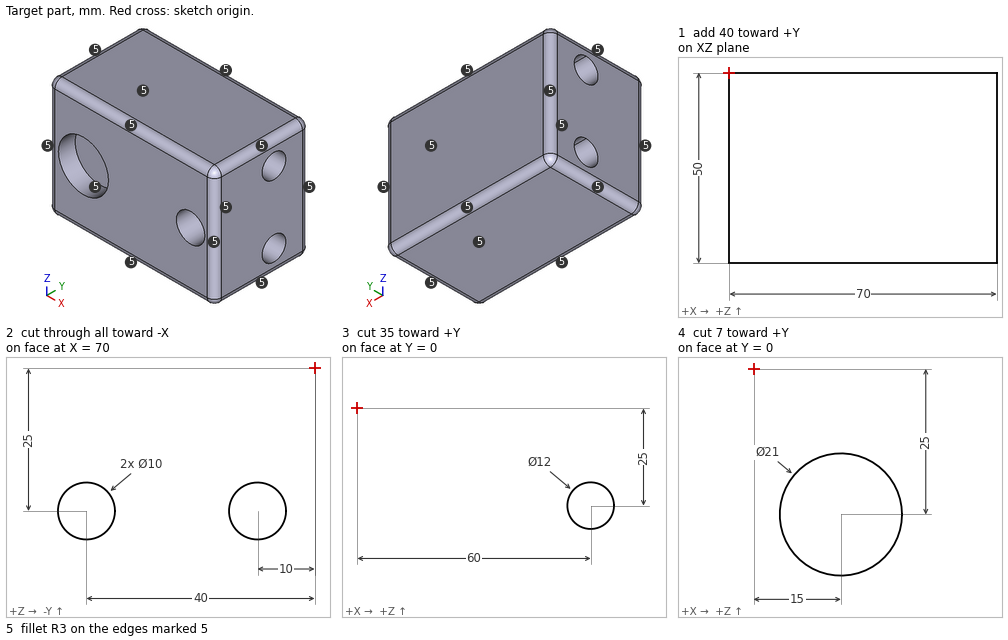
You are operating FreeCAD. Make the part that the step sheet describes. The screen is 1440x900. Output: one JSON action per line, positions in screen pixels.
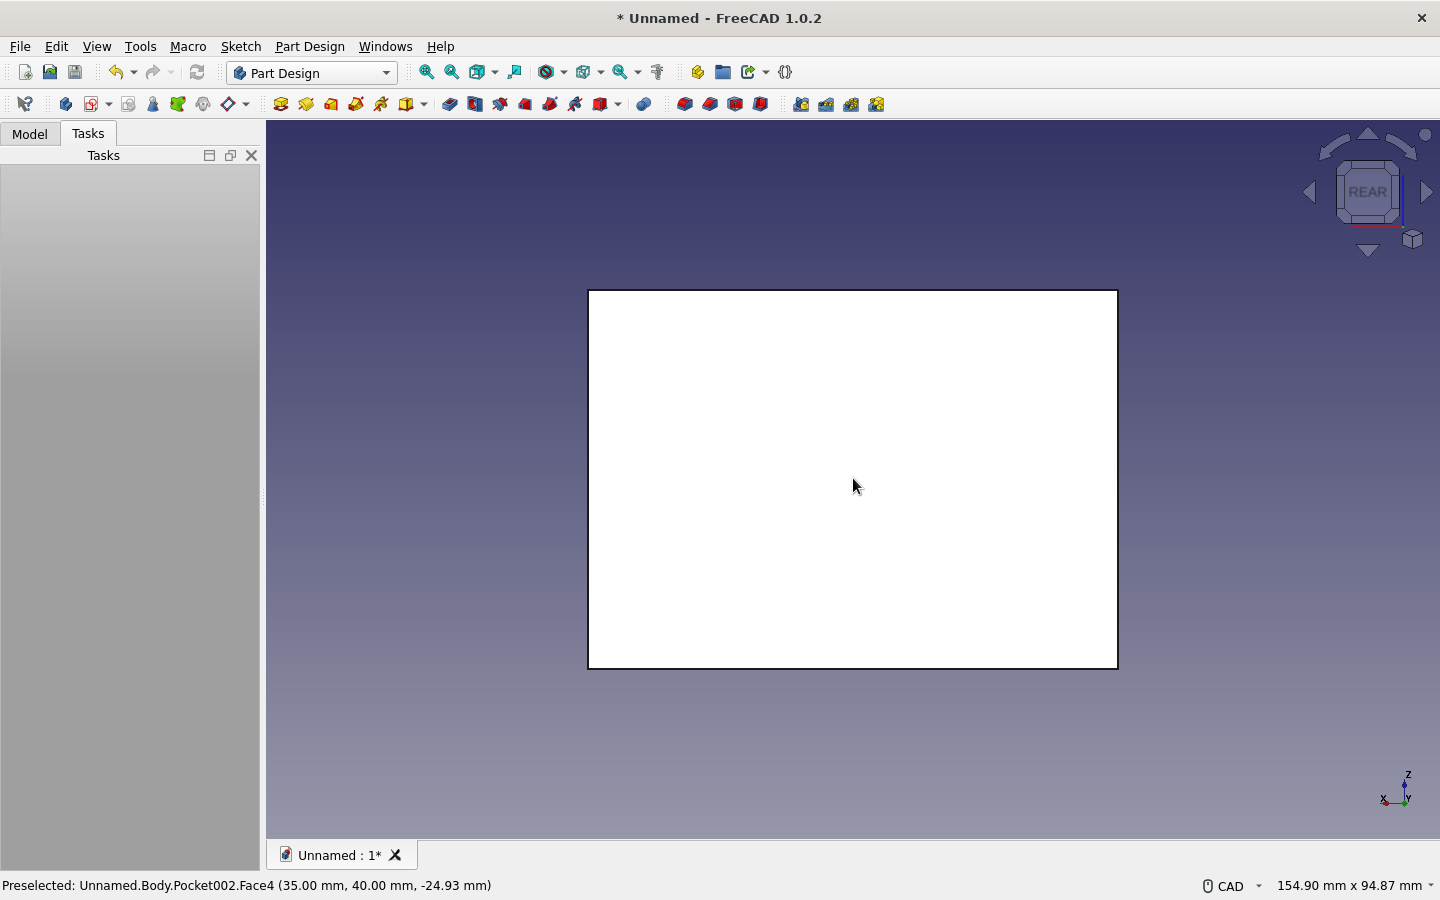
{"action": "key", "text": "6"}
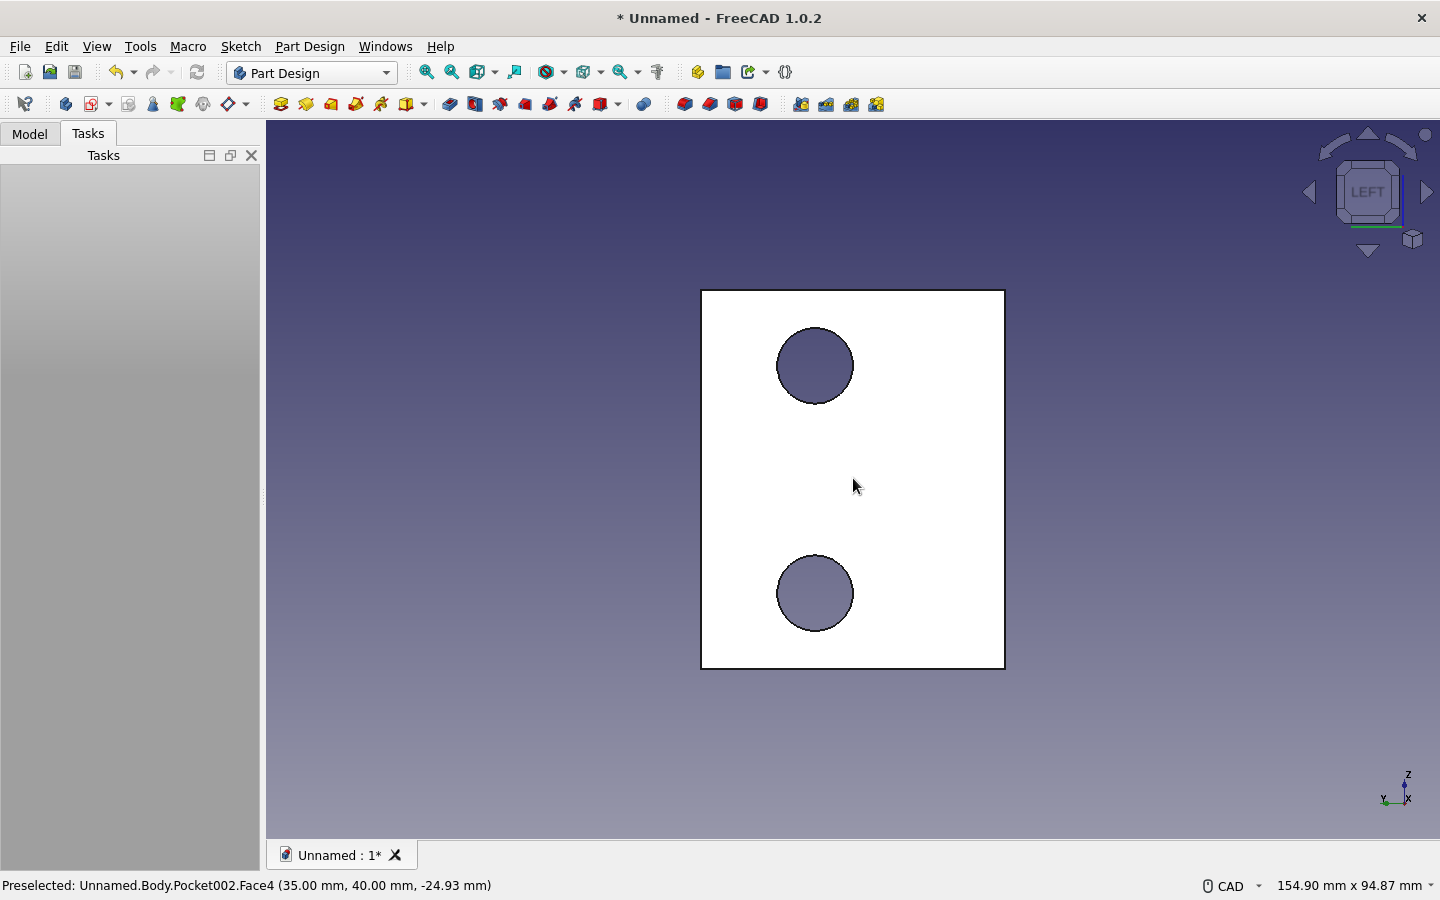
{"action": "key", "text": "v 3"}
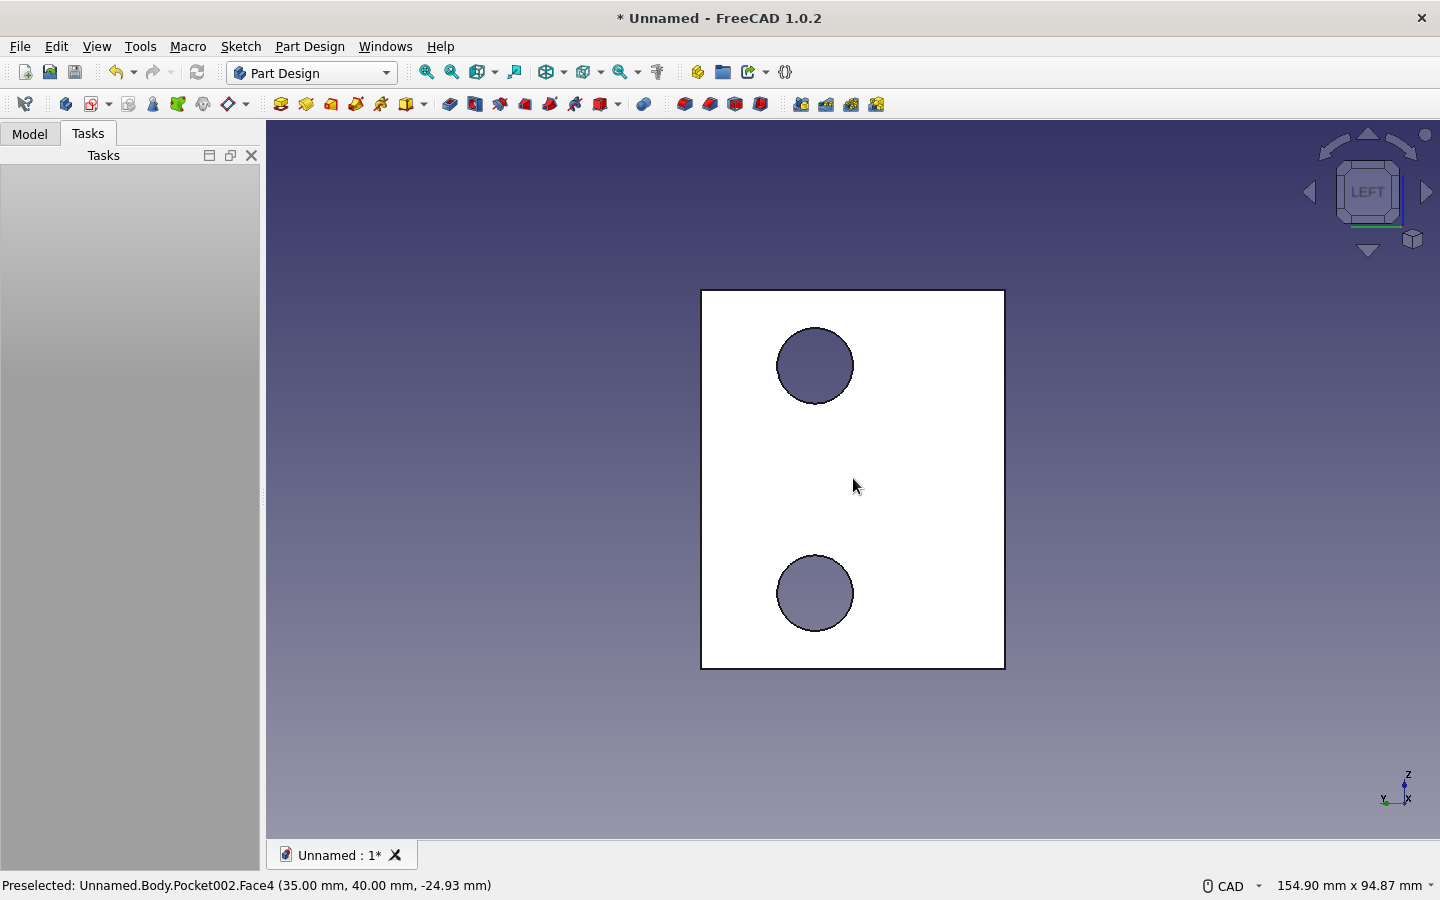
{"action": "key", "text": "0"}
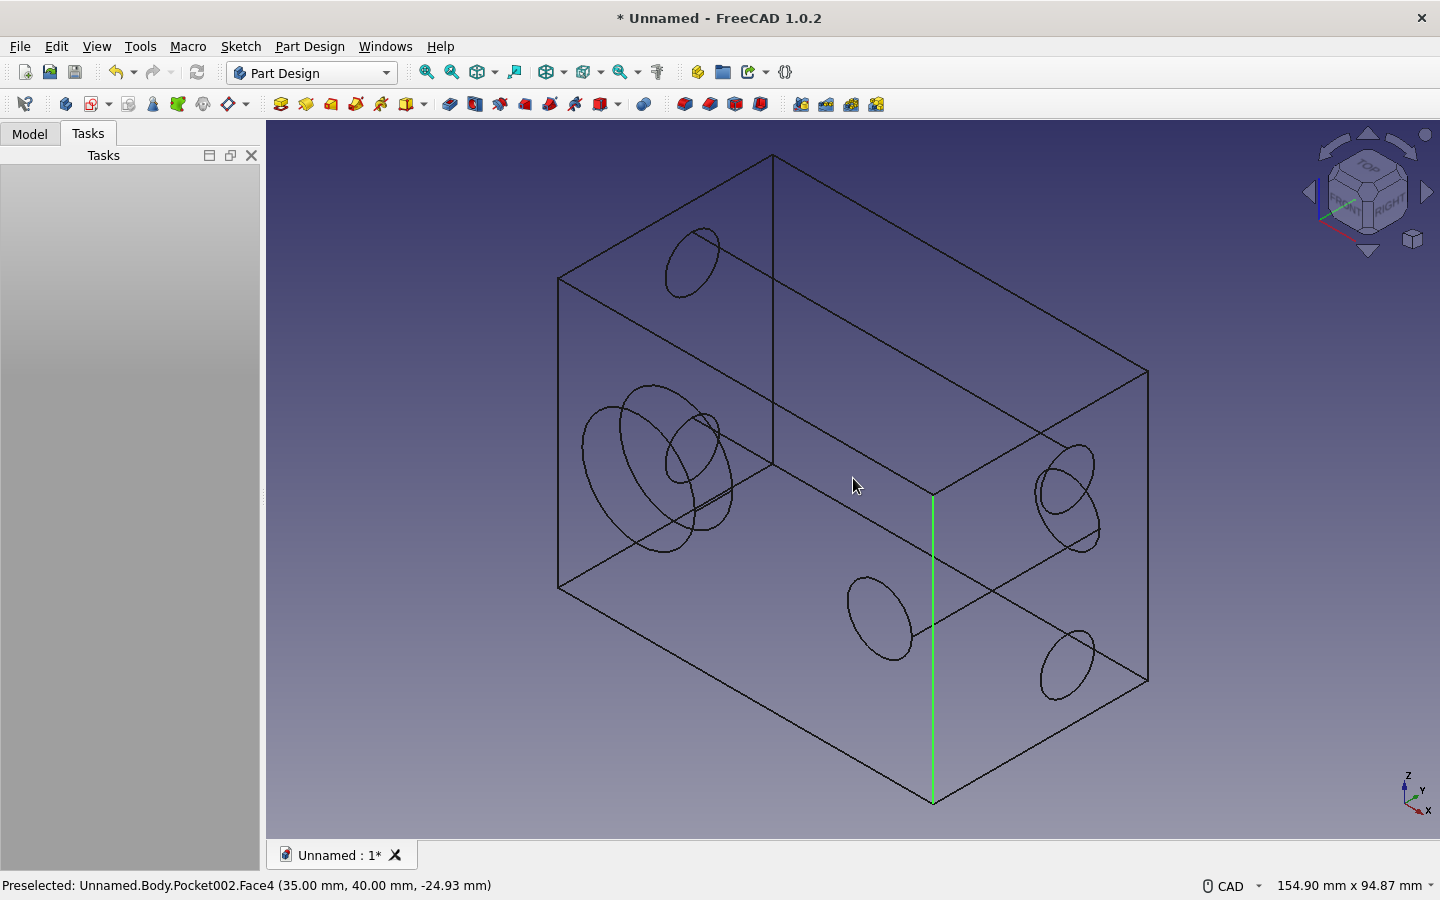
{"action": "left_click", "coordinate": [558, 432], "text": "ctrl"}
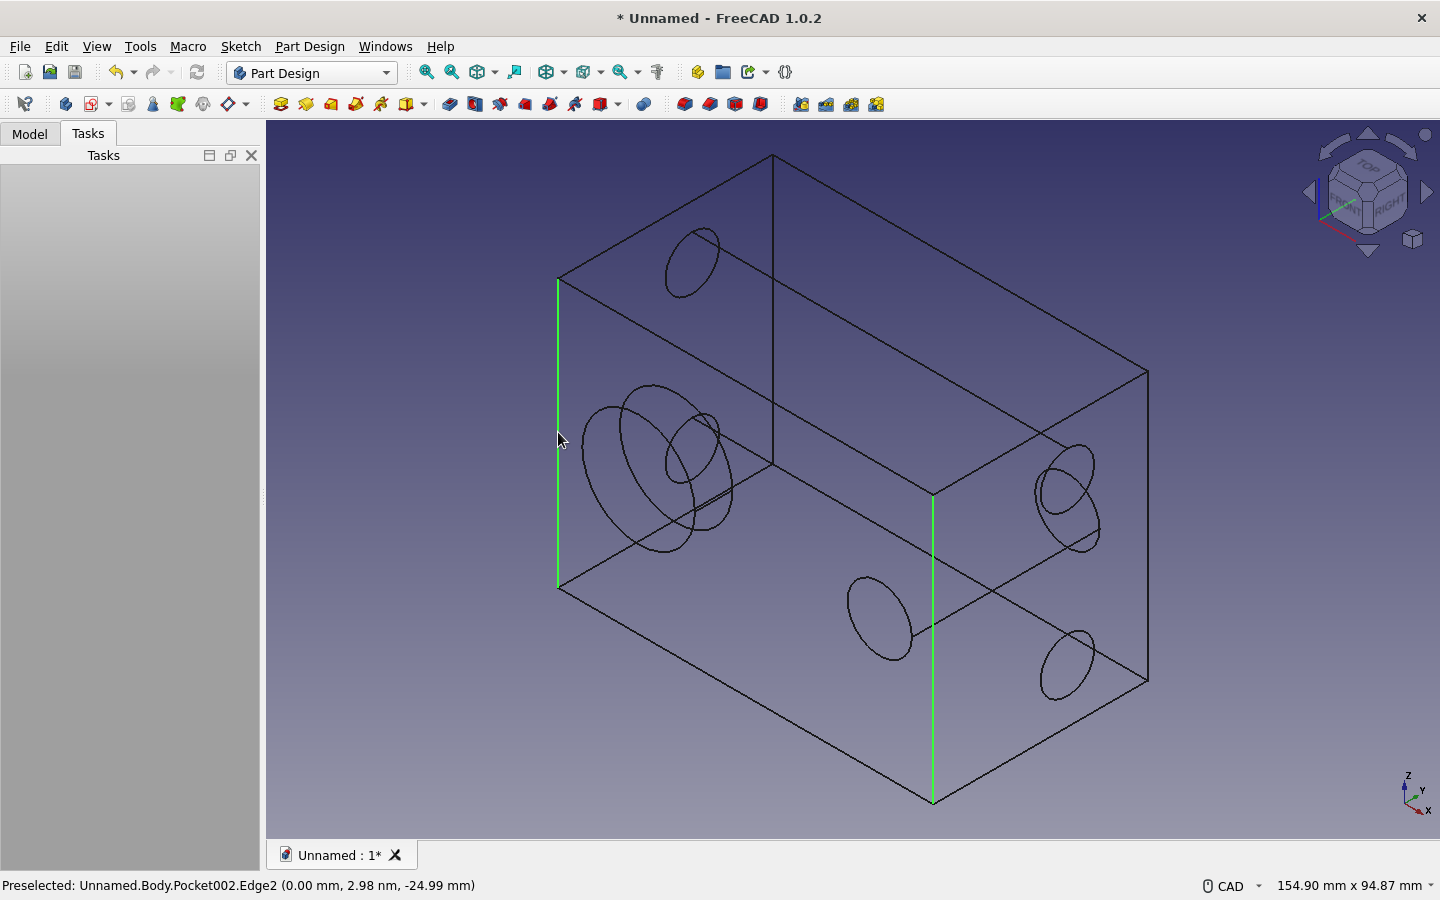
{"action": "key", "text": "v 1"}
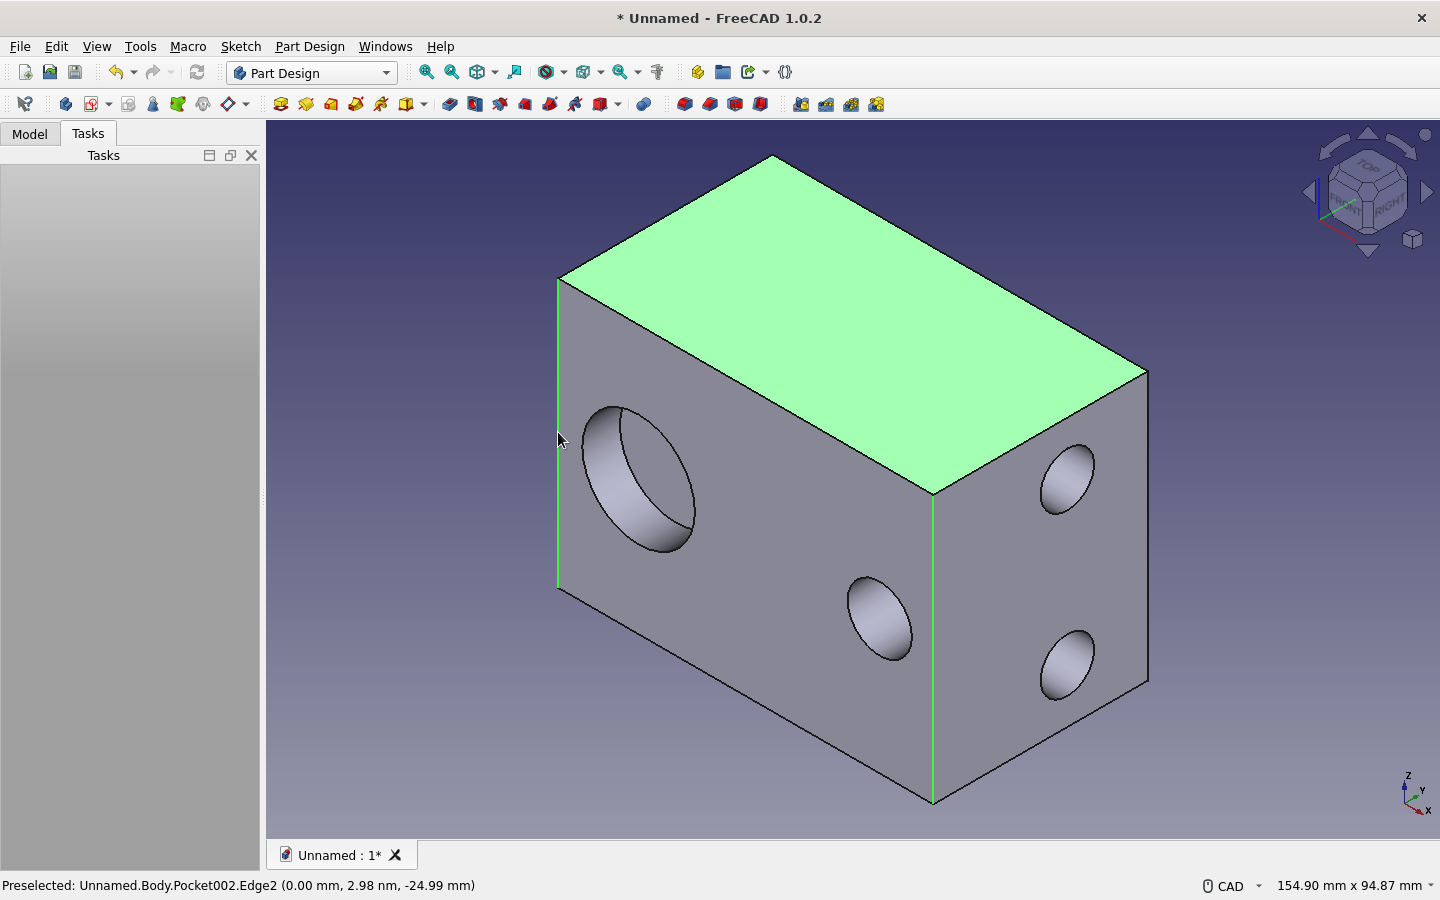
{"action": "left_click", "coordinate": [685, 104]}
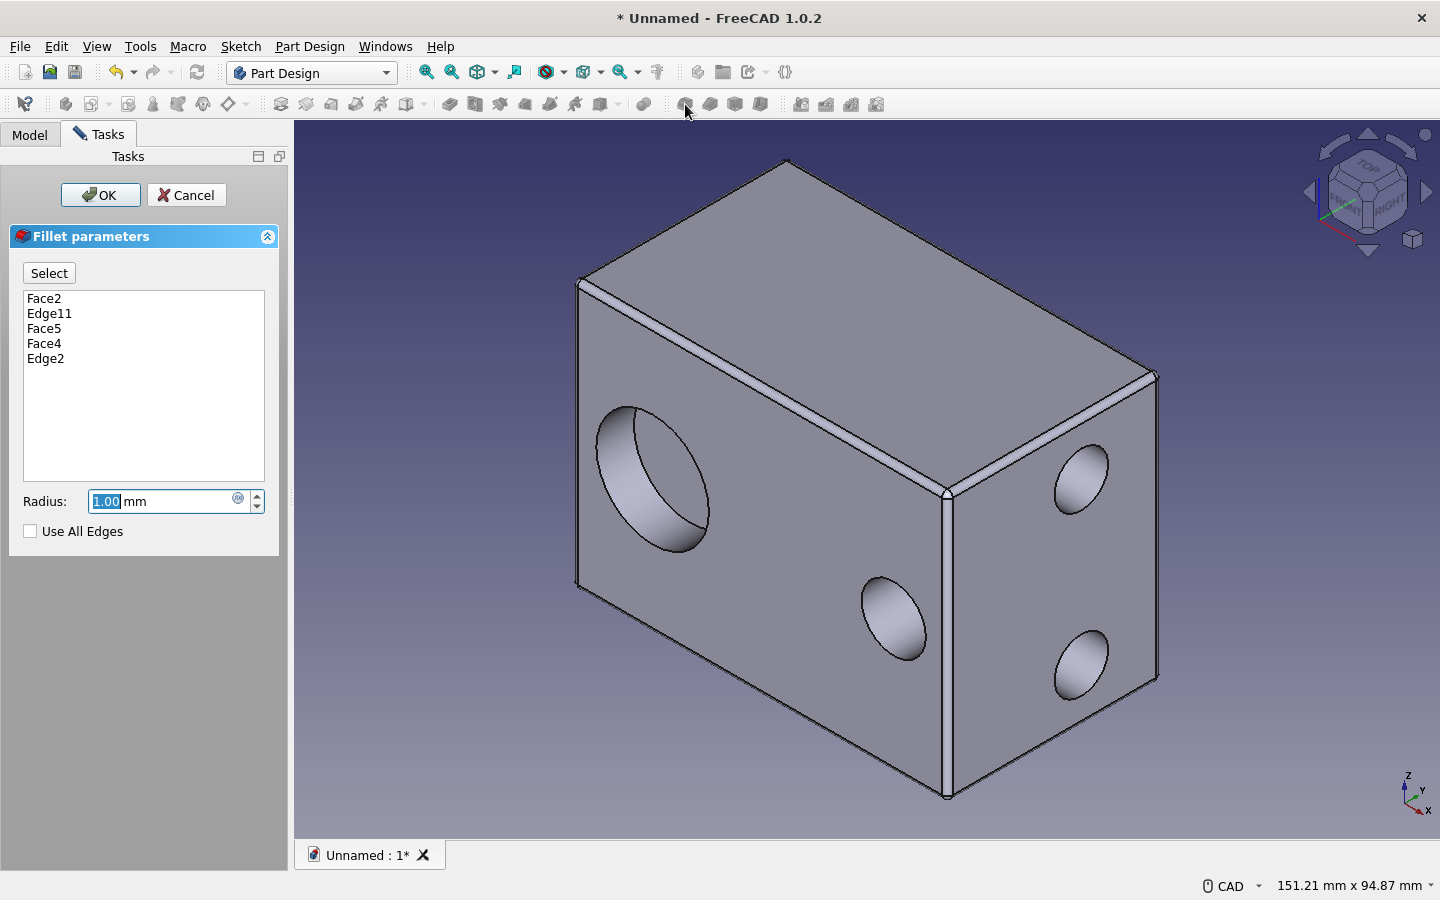
{"action": "type", "text": "3"}
{"action": "key", "text": "Tab"}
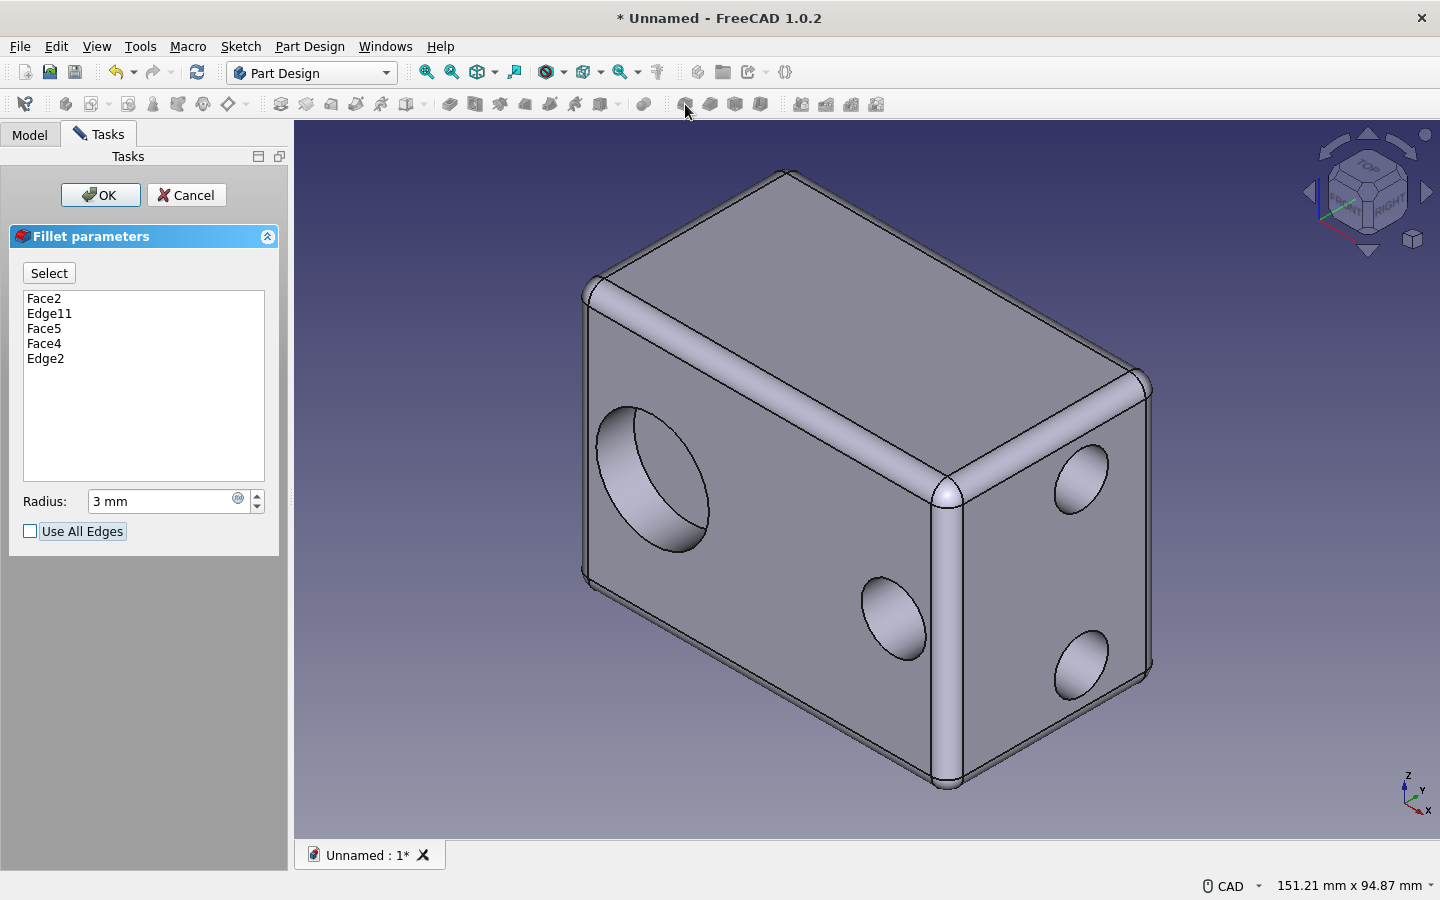
{"action": "left_click", "coordinate": [101, 195]}